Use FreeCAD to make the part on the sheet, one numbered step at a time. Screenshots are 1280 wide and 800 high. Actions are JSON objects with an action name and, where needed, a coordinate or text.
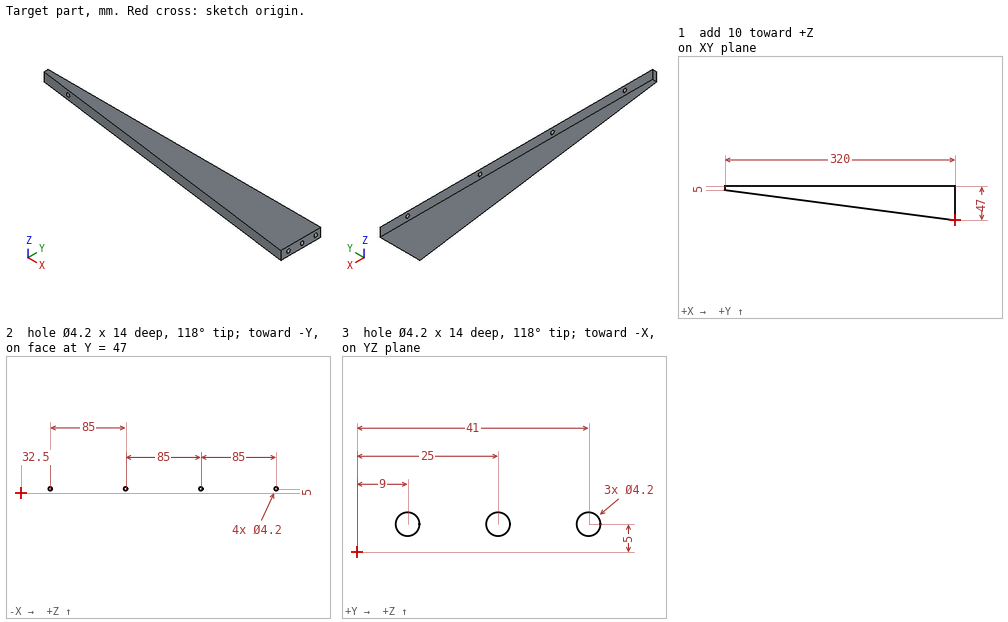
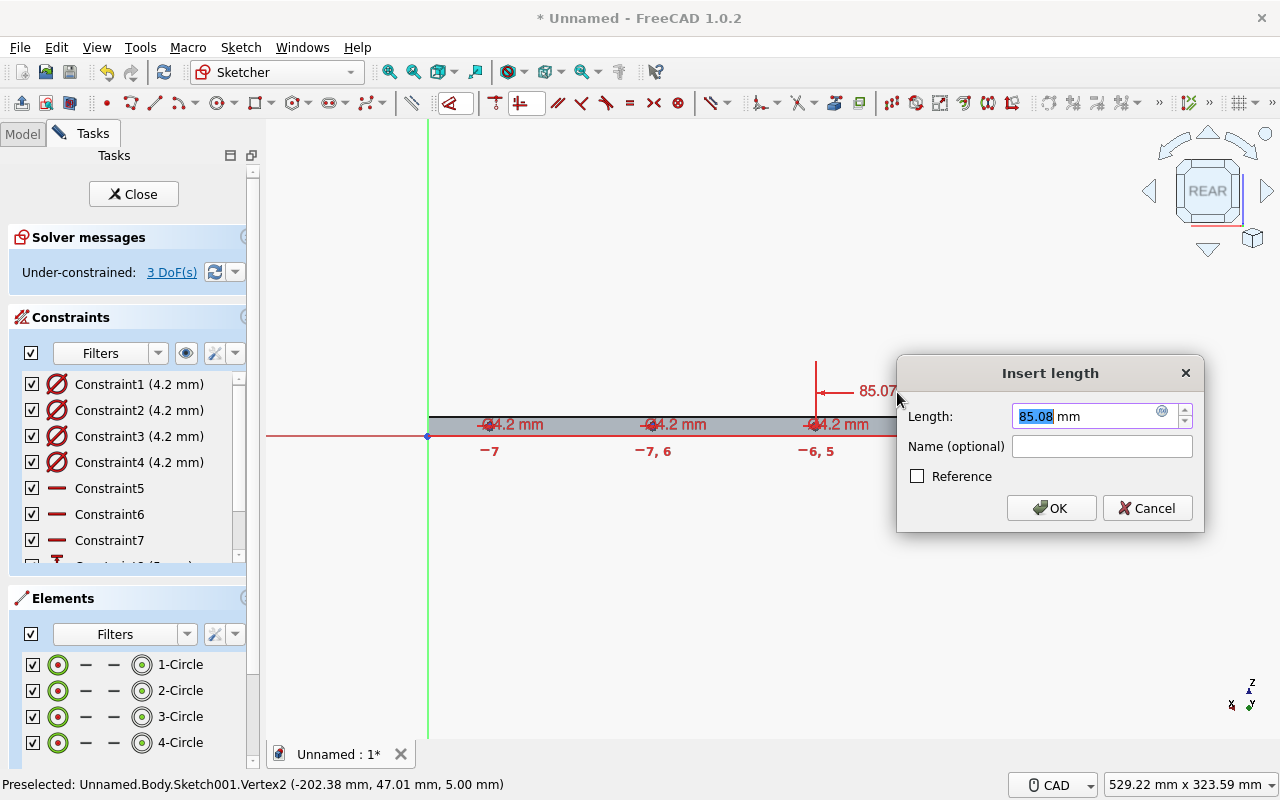
{"action": "type", "text": "85"}
{"action": "key", "text": "Return"}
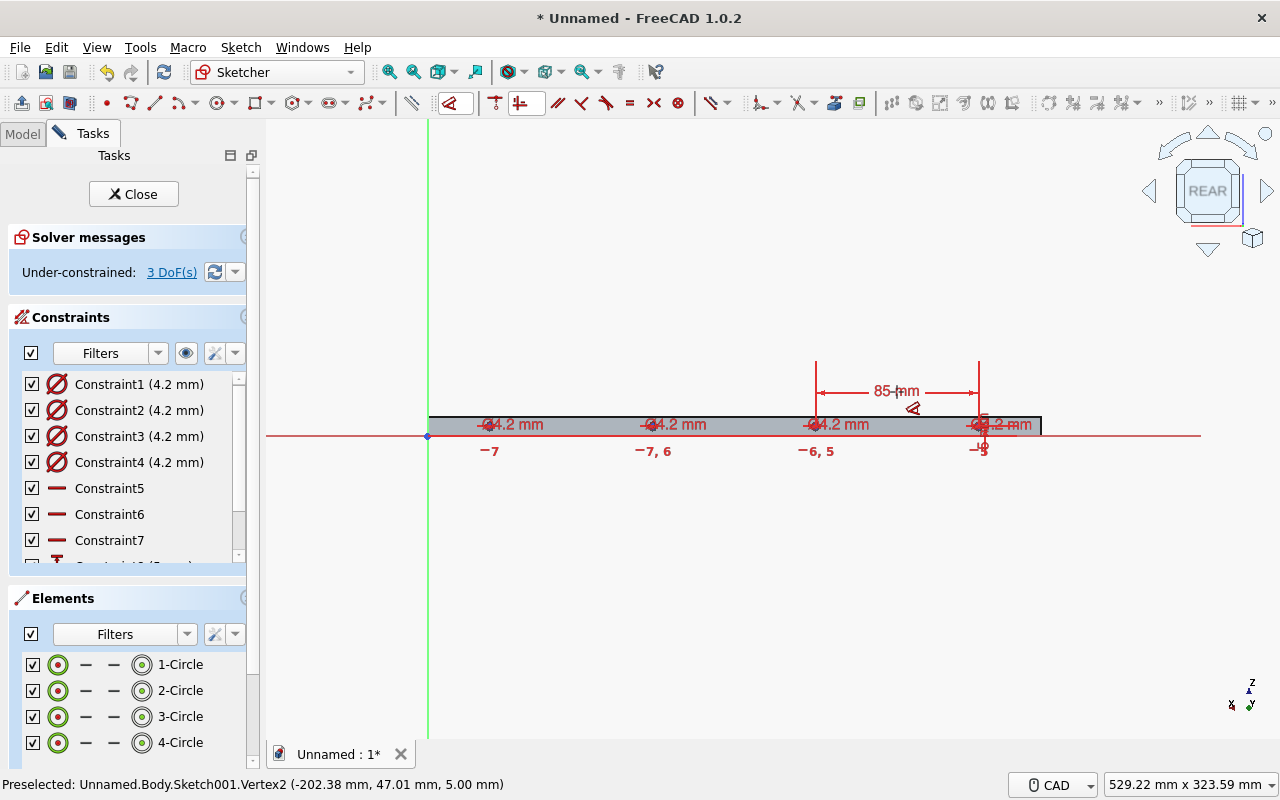
{"action": "left_click", "coordinate": [816, 426]}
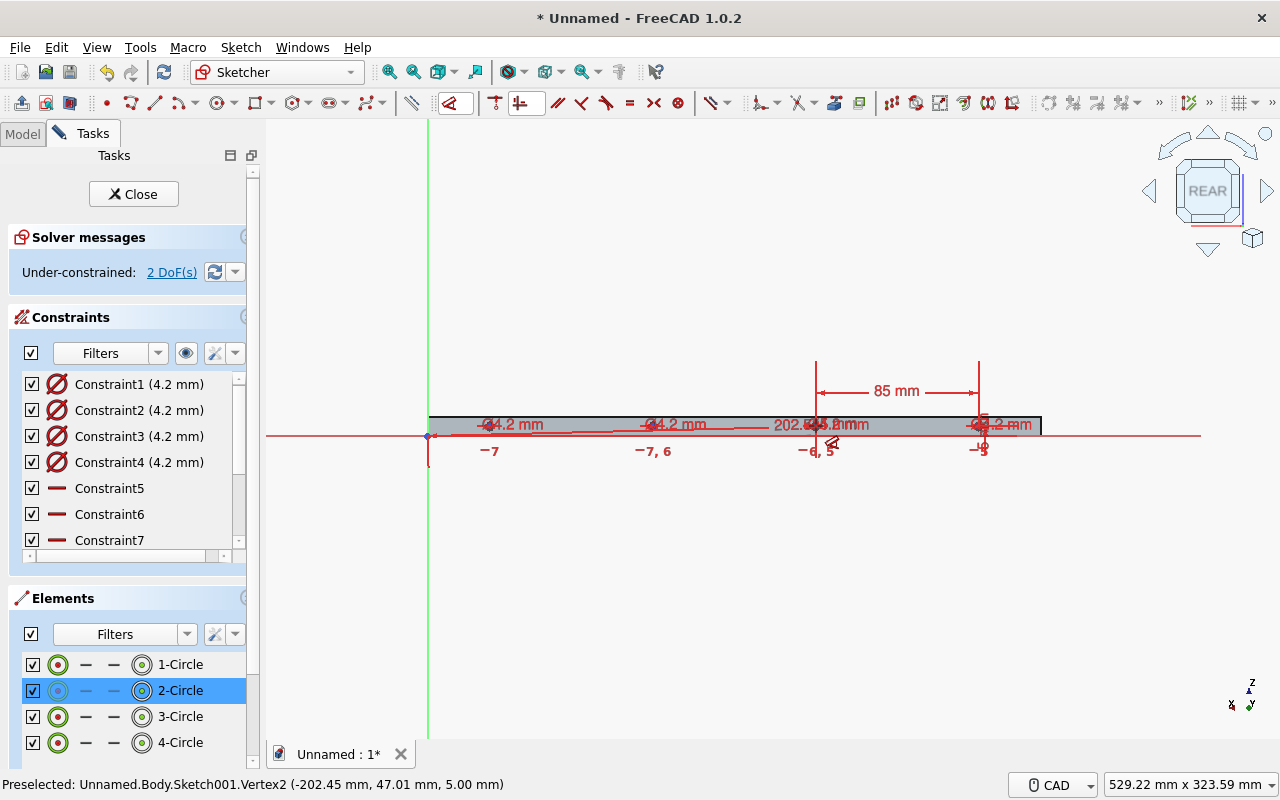
{"action": "left_click", "coordinate": [653, 426]}
{"action": "left_click", "coordinate": [734, 392]}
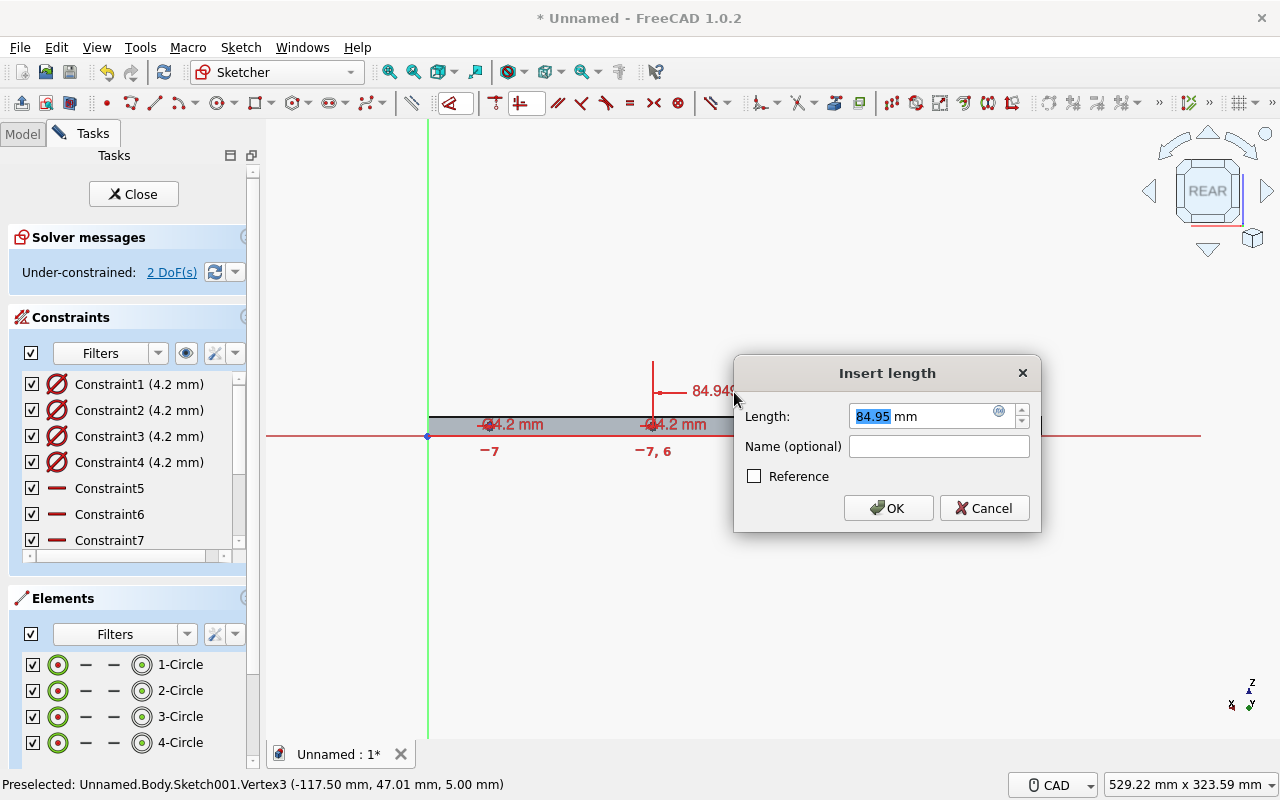
{"action": "type", "text": "85"}
{"action": "key", "text": "Return"}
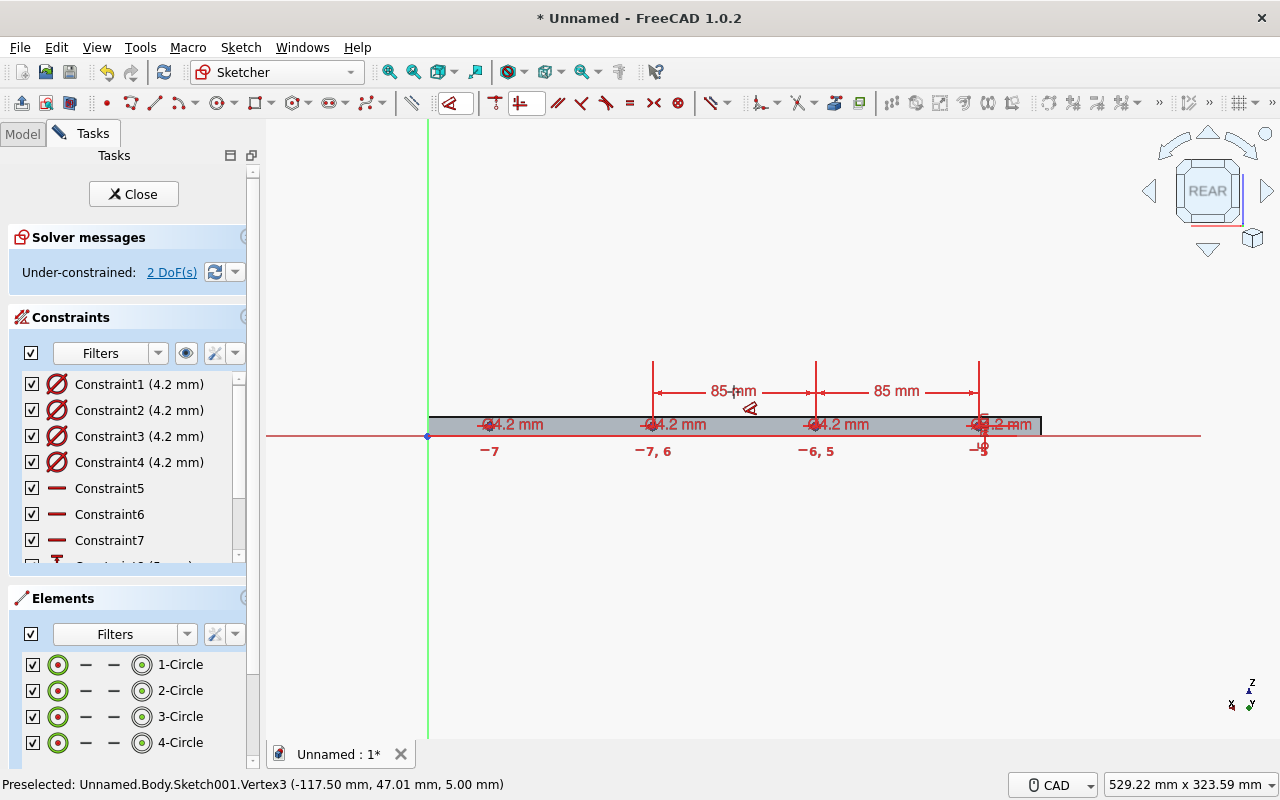
{"action": "left_click", "coordinate": [653, 426]}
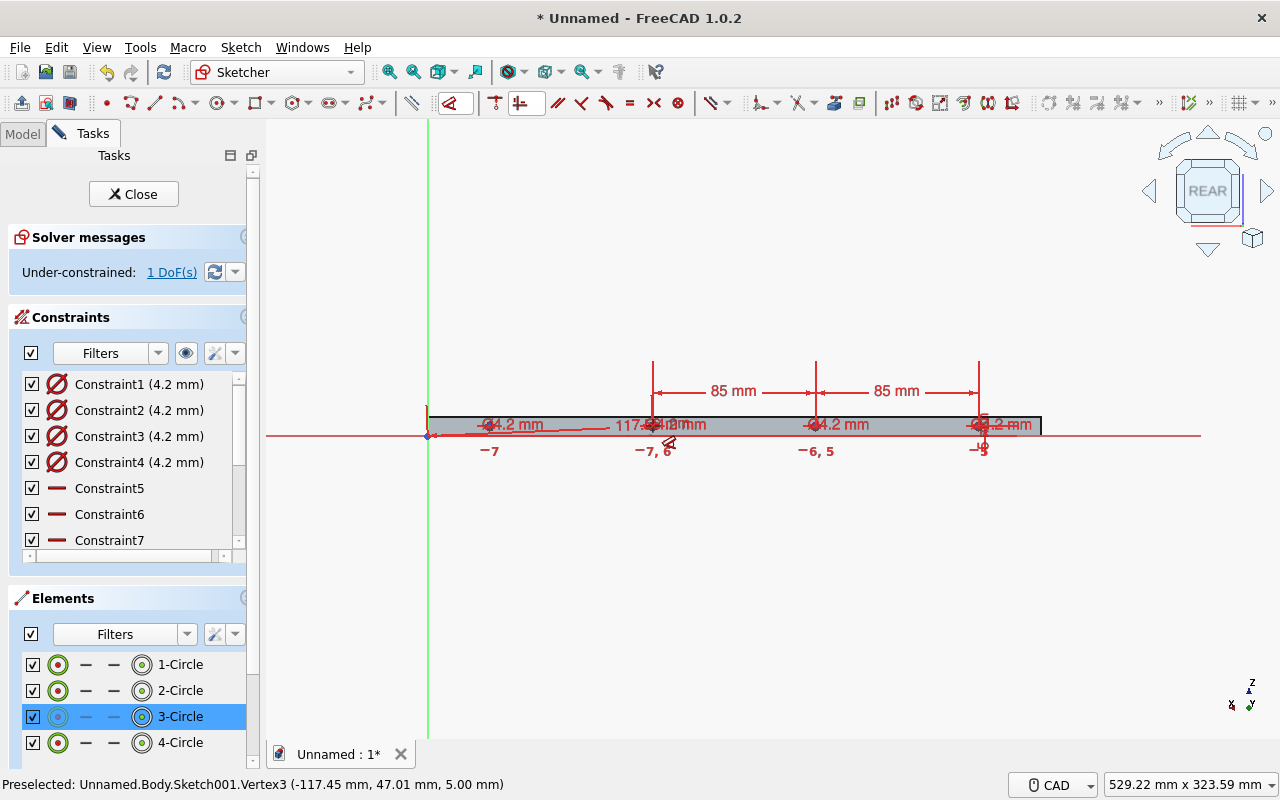
{"action": "left_click", "coordinate": [490, 426]}
{"action": "left_click", "coordinate": [571, 392]}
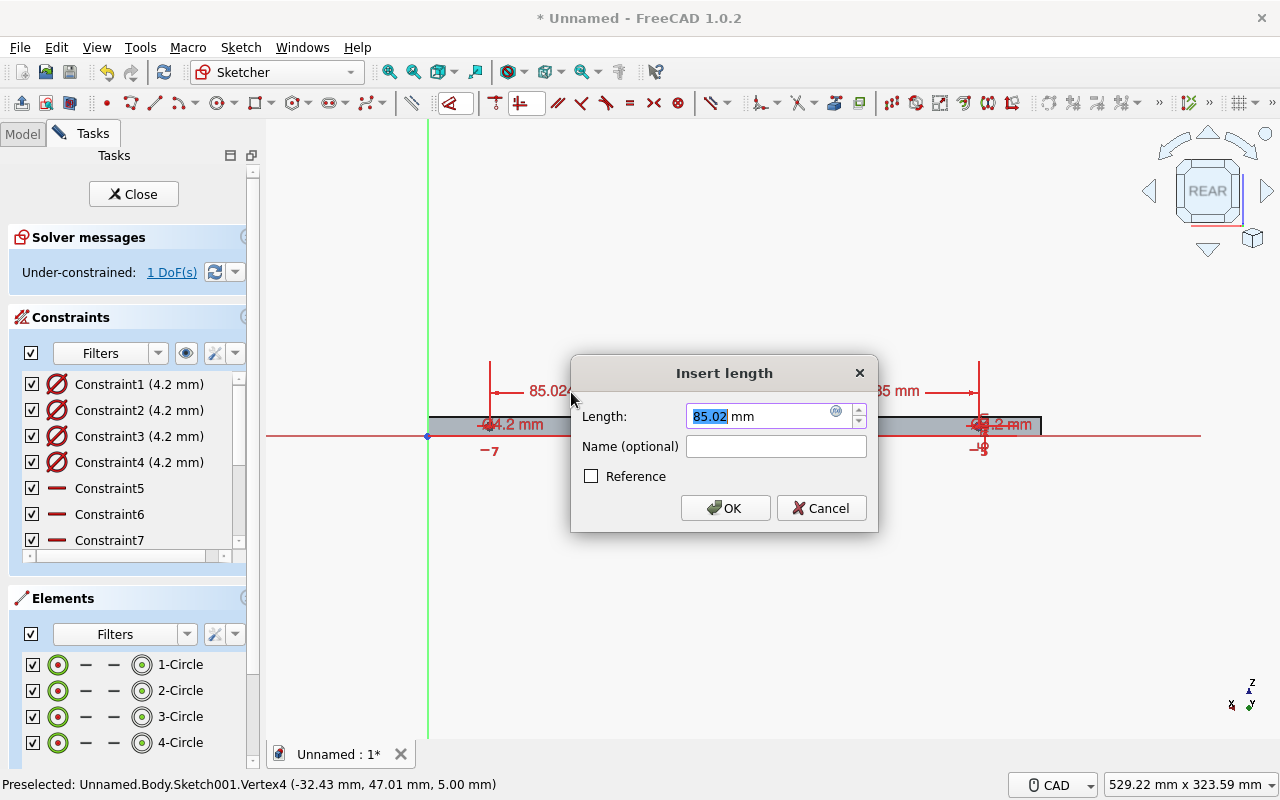
{"action": "type", "text": "85"}
{"action": "key", "text": "Return"}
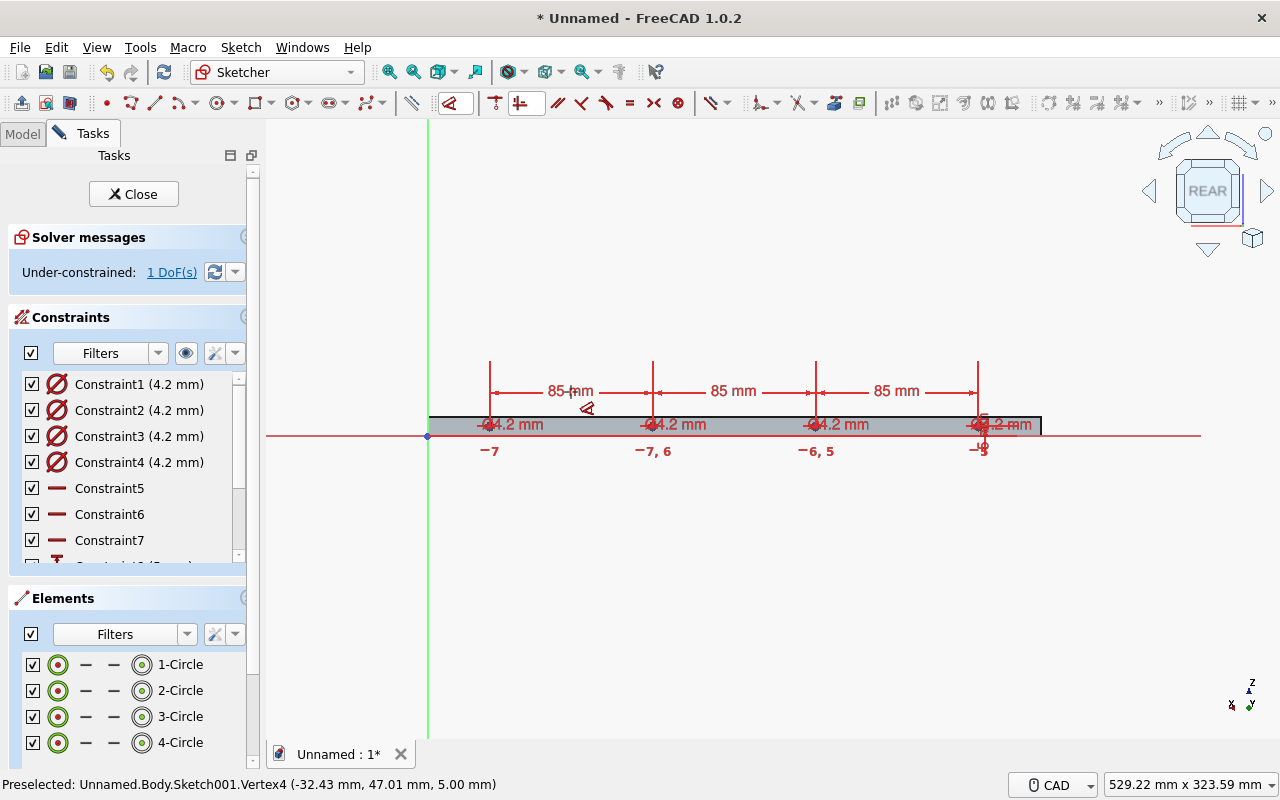
{"action": "left_click", "coordinate": [490, 426]}
{"action": "left_click", "coordinate": [459, 470]}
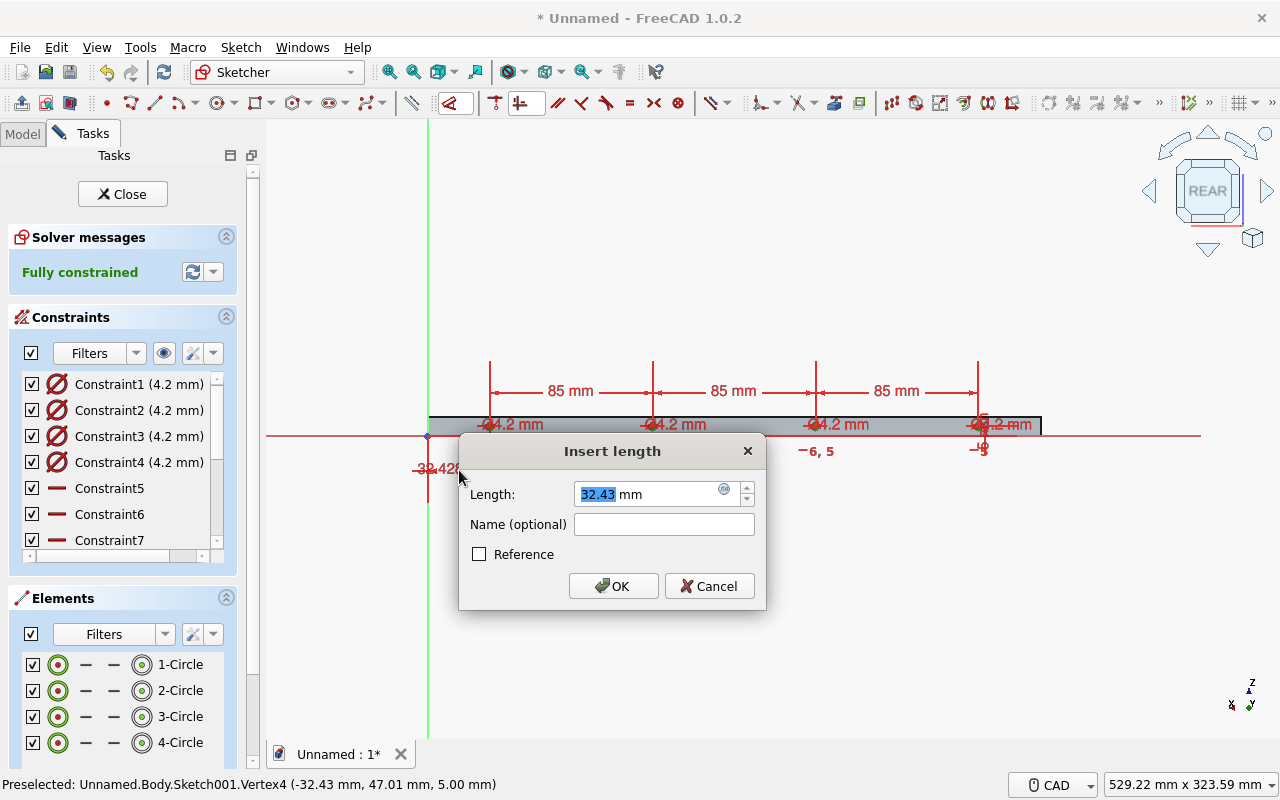
{"action": "type", "text": "32.5"}
{"action": "key", "text": "Return"}
{"action": "key", "text": "Escape"}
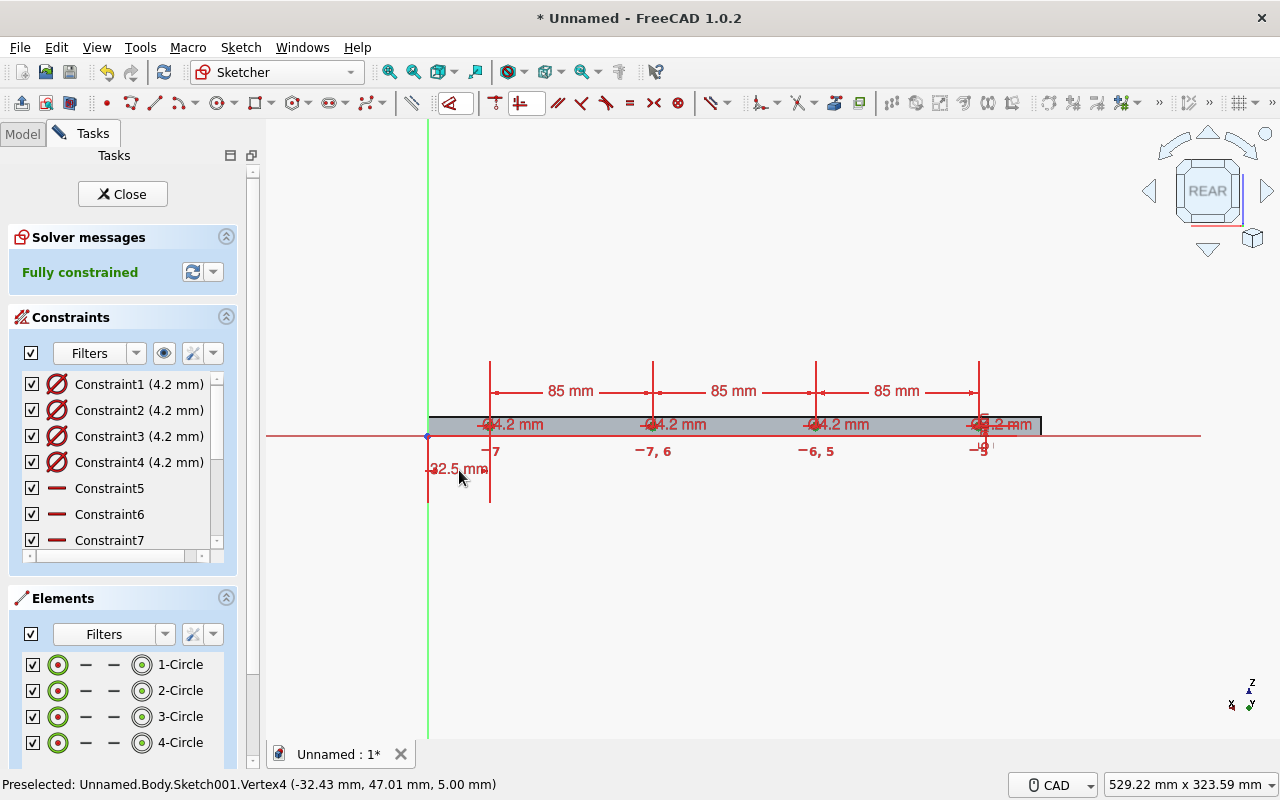
{"action": "left_click", "coordinate": [123, 194]}